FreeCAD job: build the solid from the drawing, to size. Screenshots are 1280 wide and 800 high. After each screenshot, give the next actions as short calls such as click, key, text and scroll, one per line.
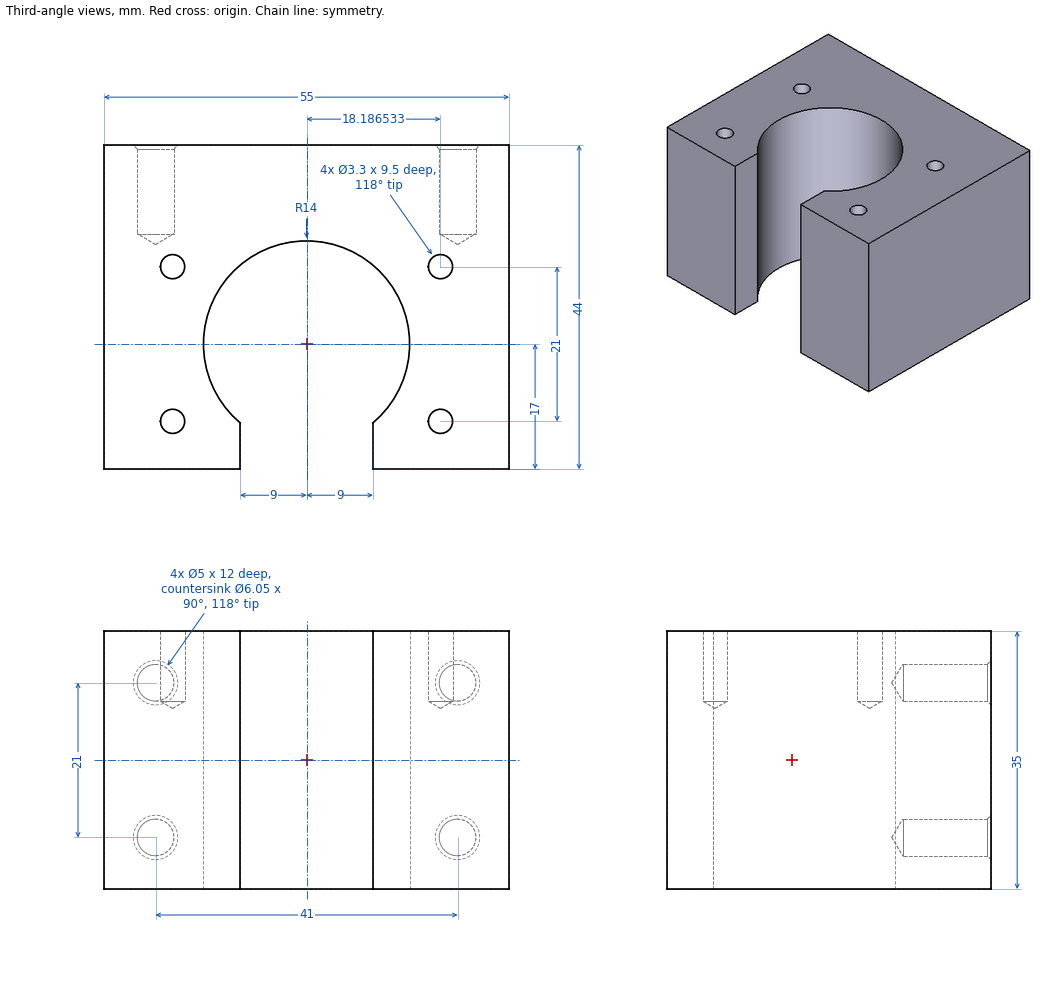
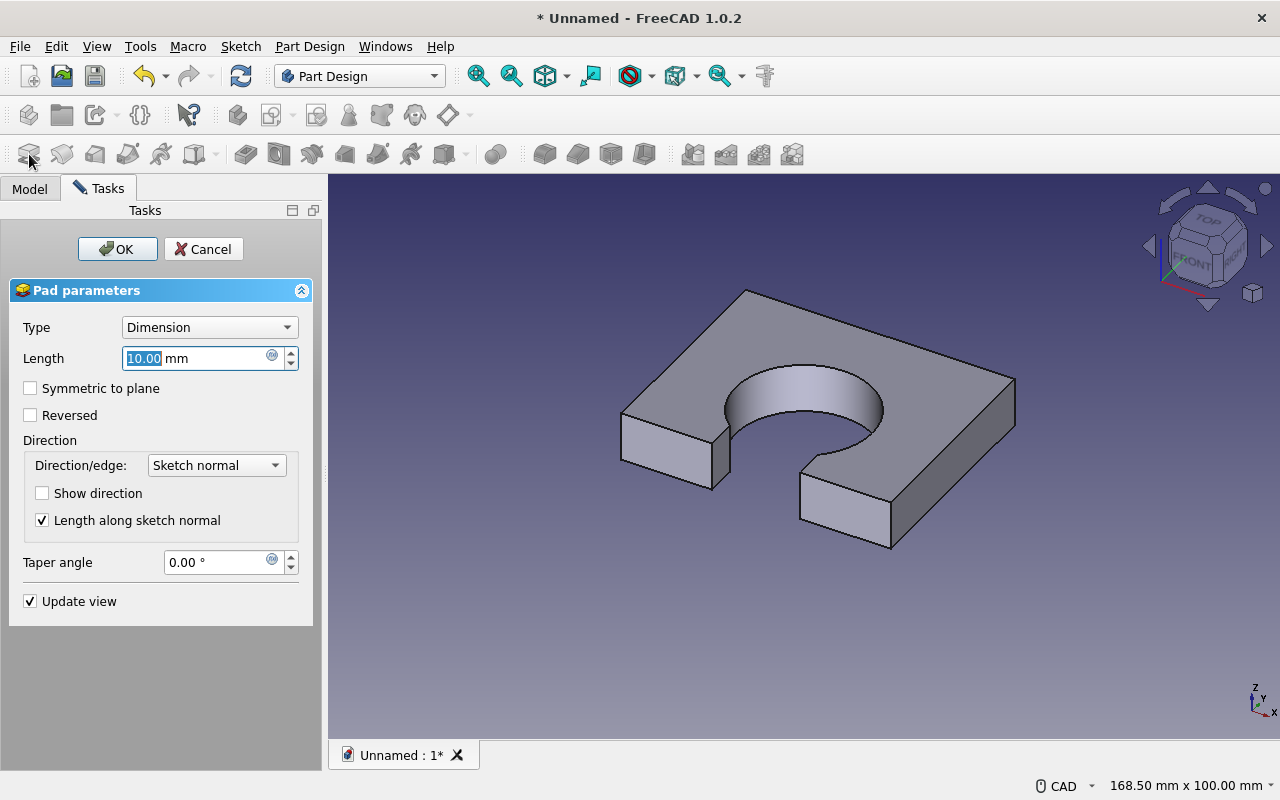
text(35)
key(Tab)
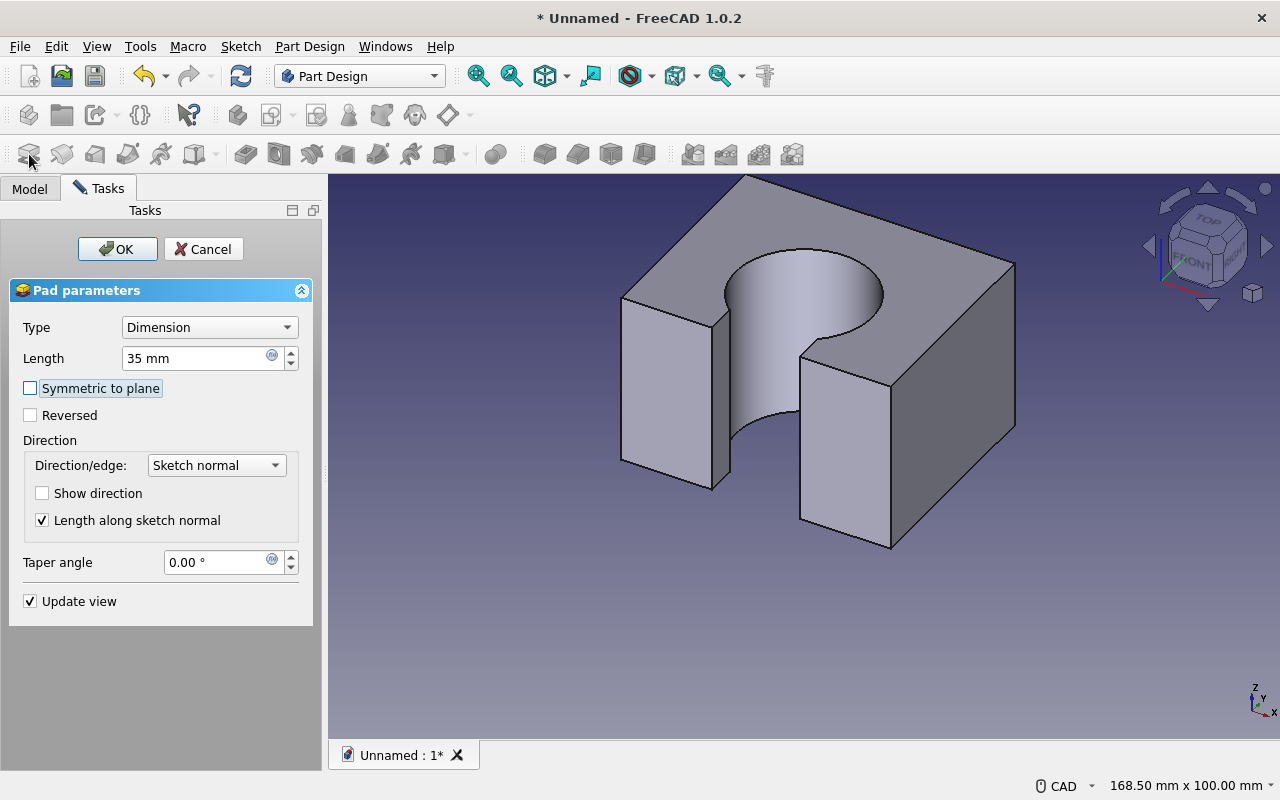
click(31, 388)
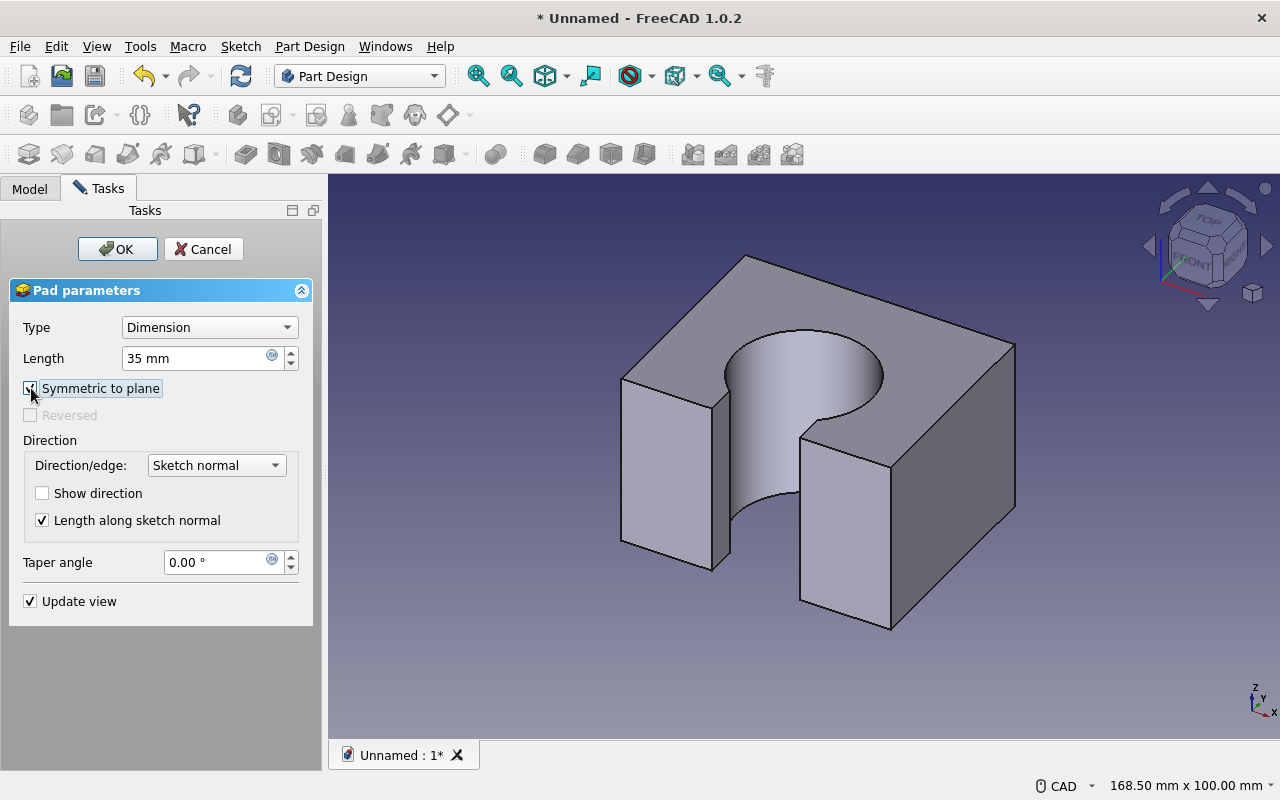
click(118, 249)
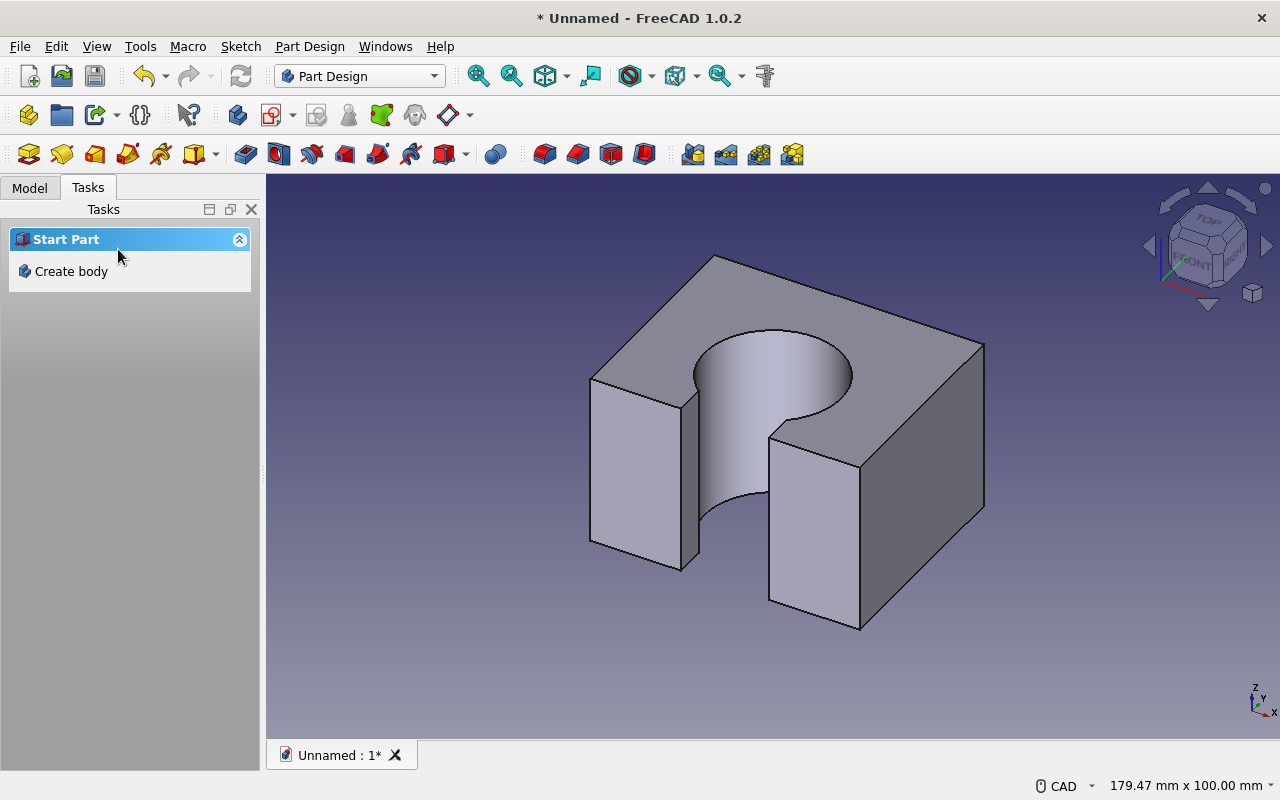
click(900, 351)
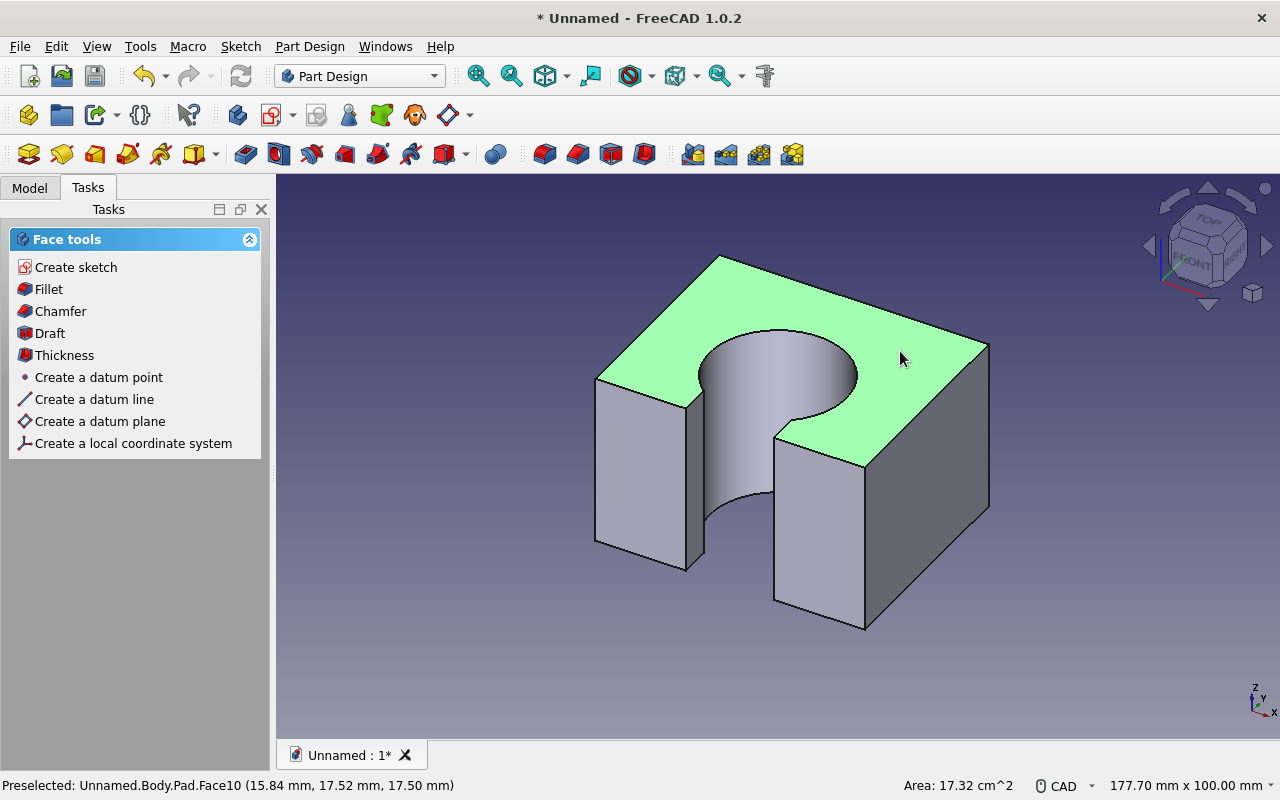
click(270, 116)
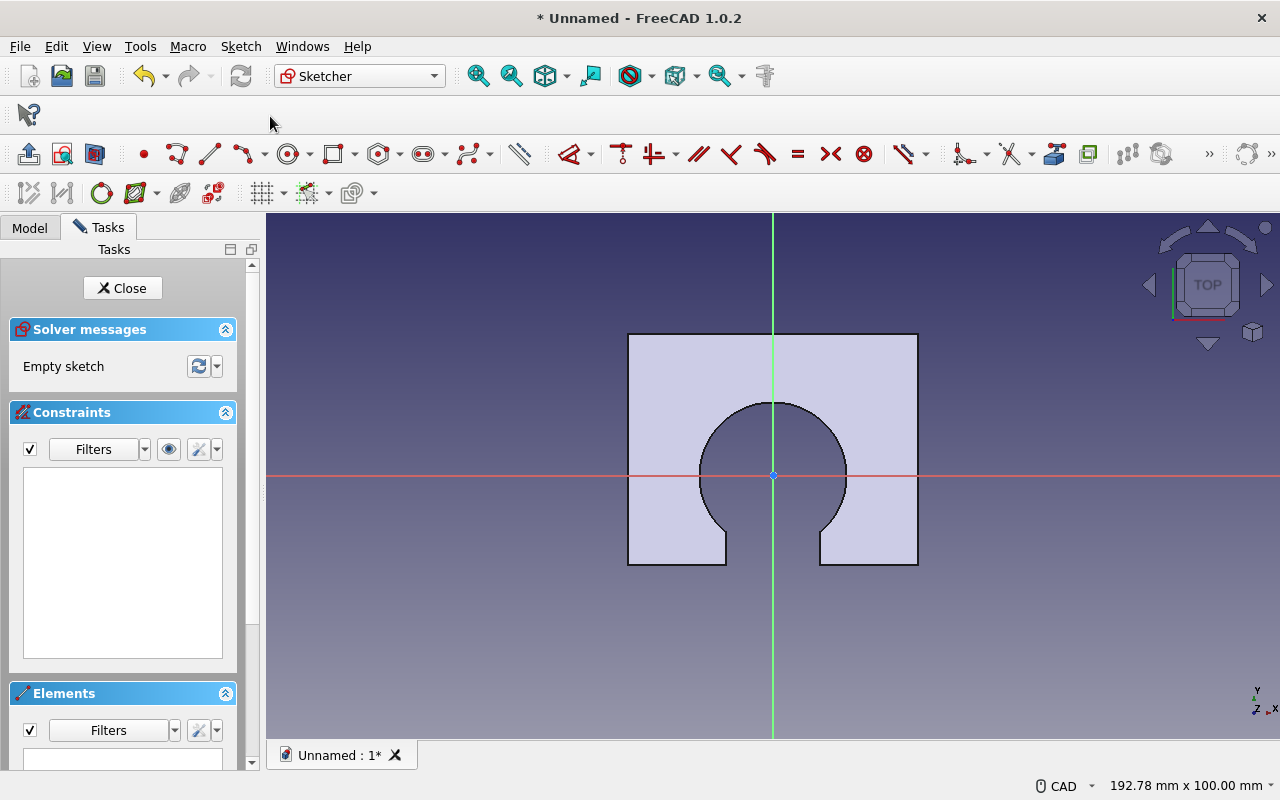
scroll(813, 476, up, 5)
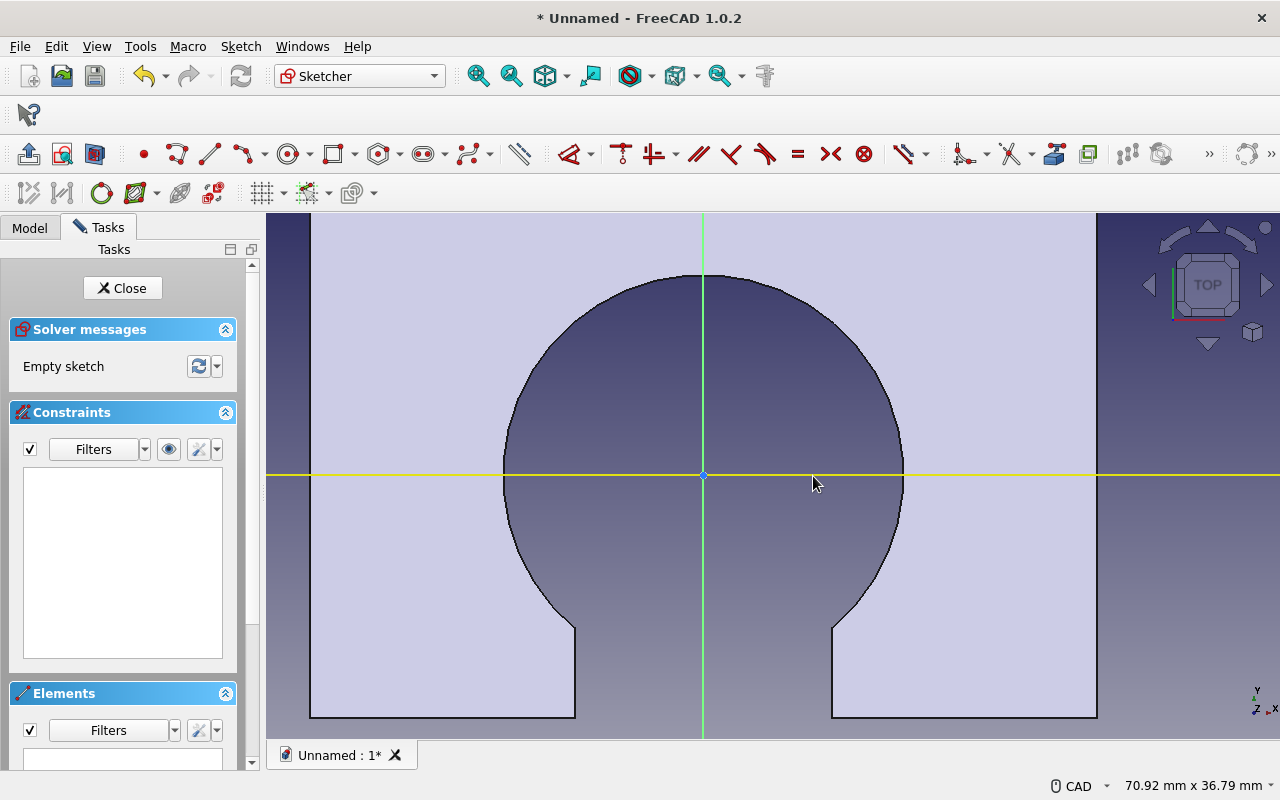
click(288, 154)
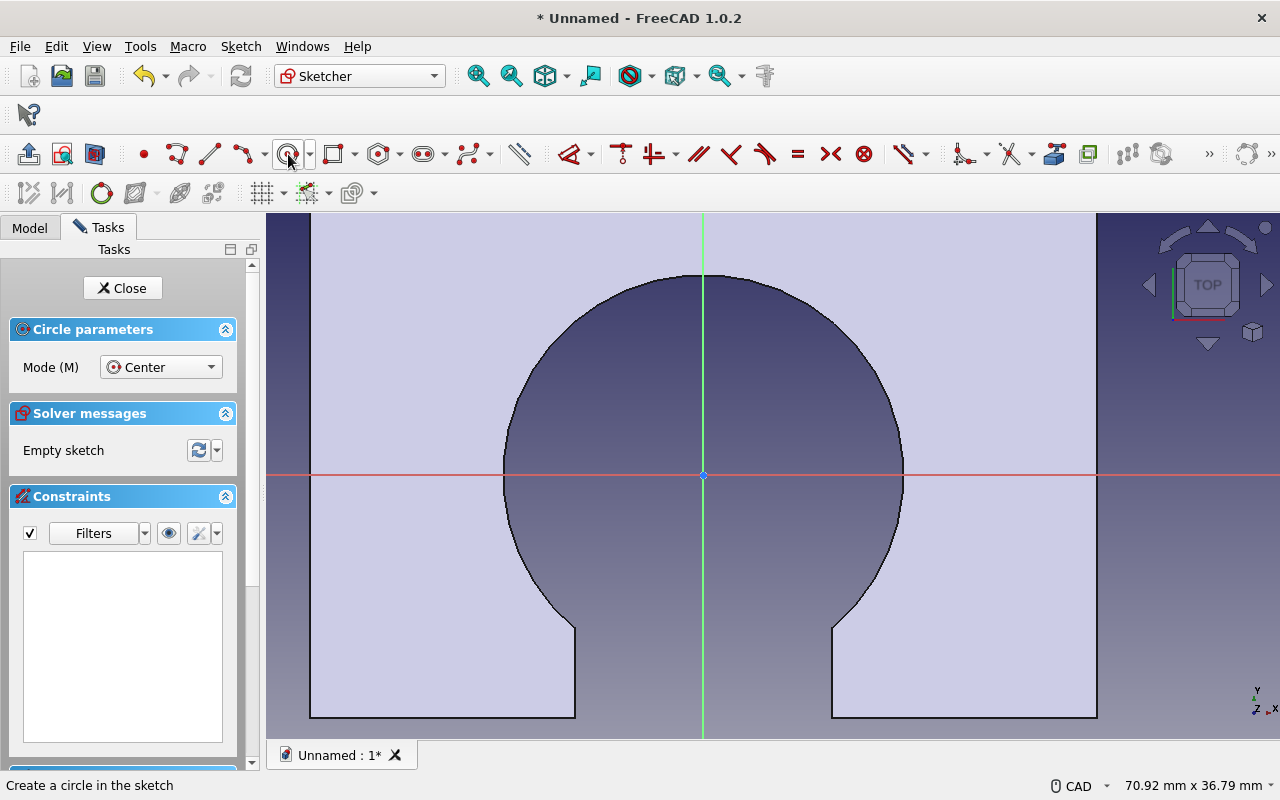
click(963, 325)
move(980, 308)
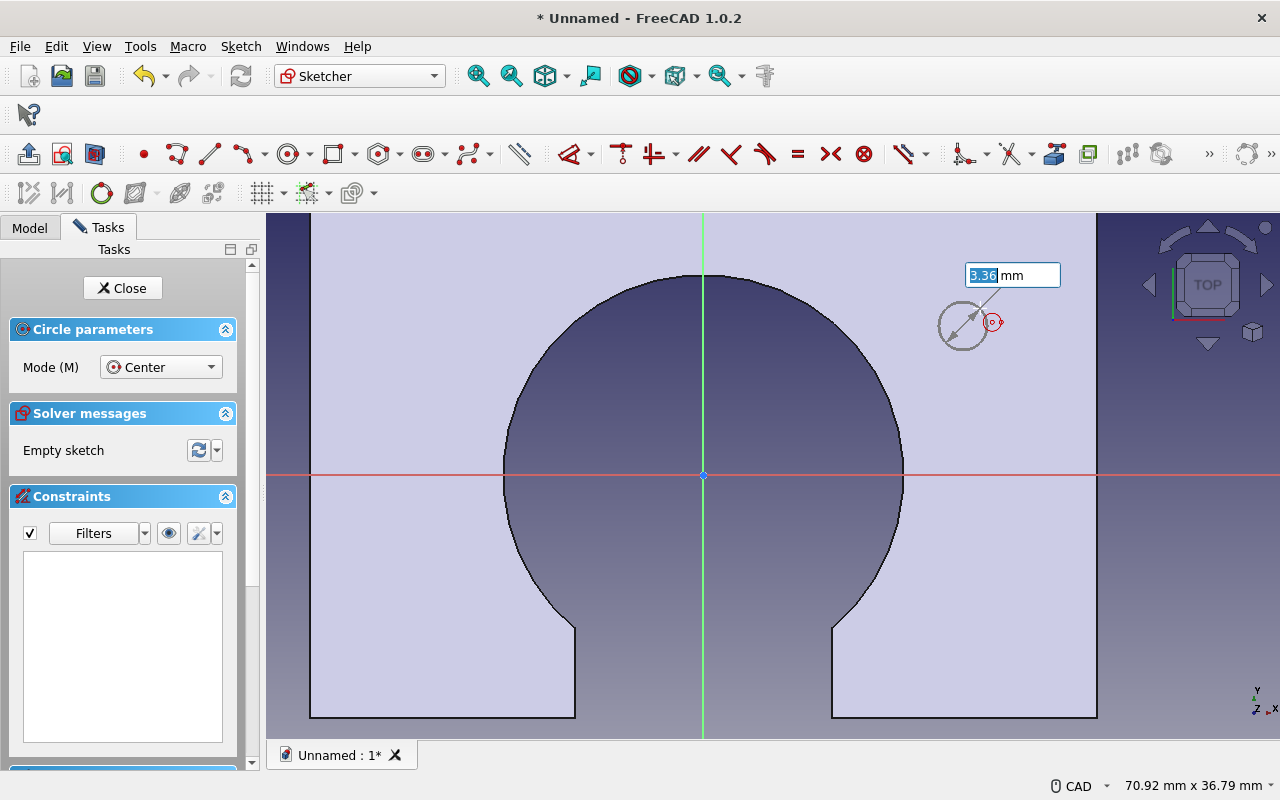
text(3.3)
key(Return)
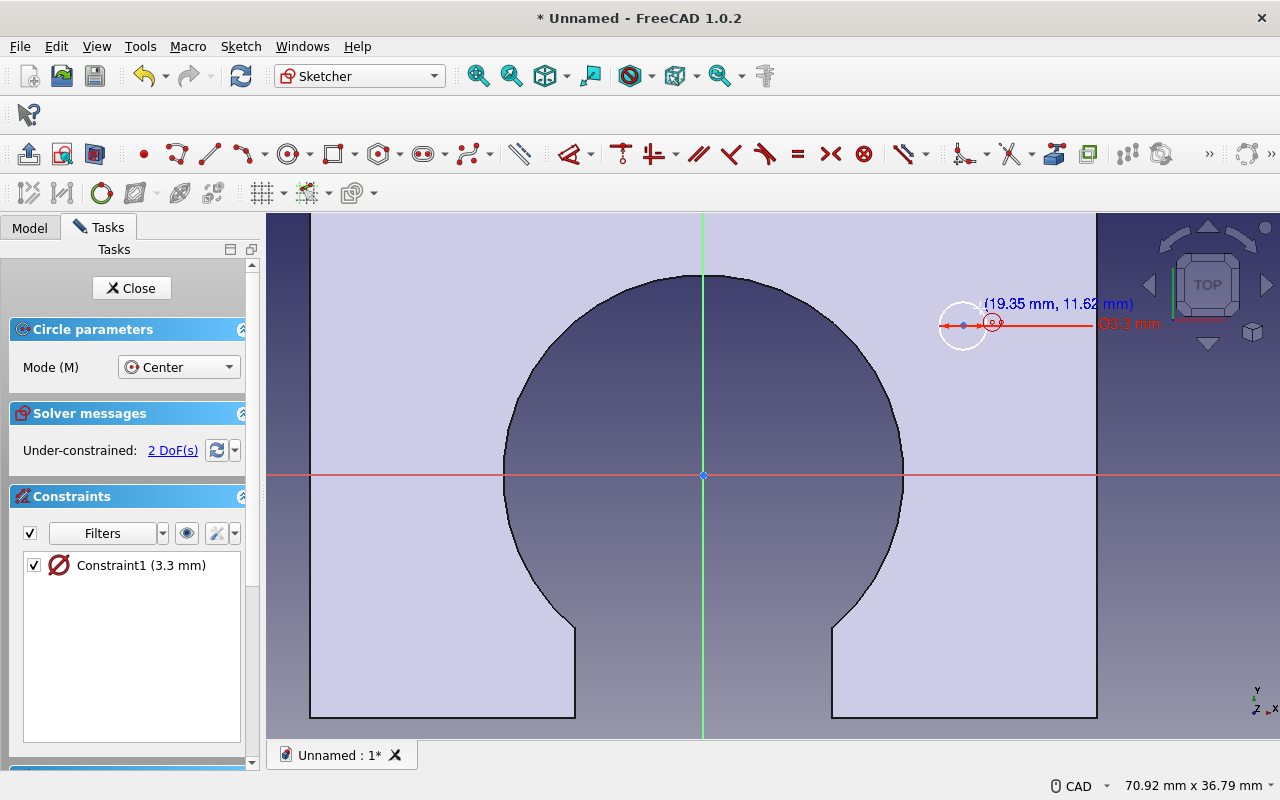
click(963, 625)
move(980, 609)